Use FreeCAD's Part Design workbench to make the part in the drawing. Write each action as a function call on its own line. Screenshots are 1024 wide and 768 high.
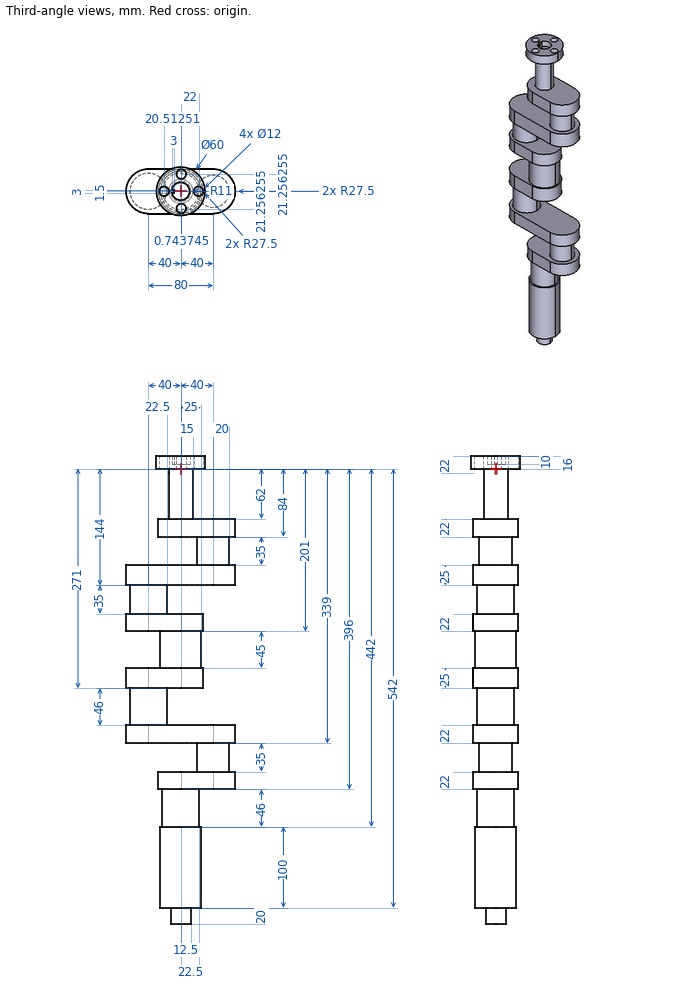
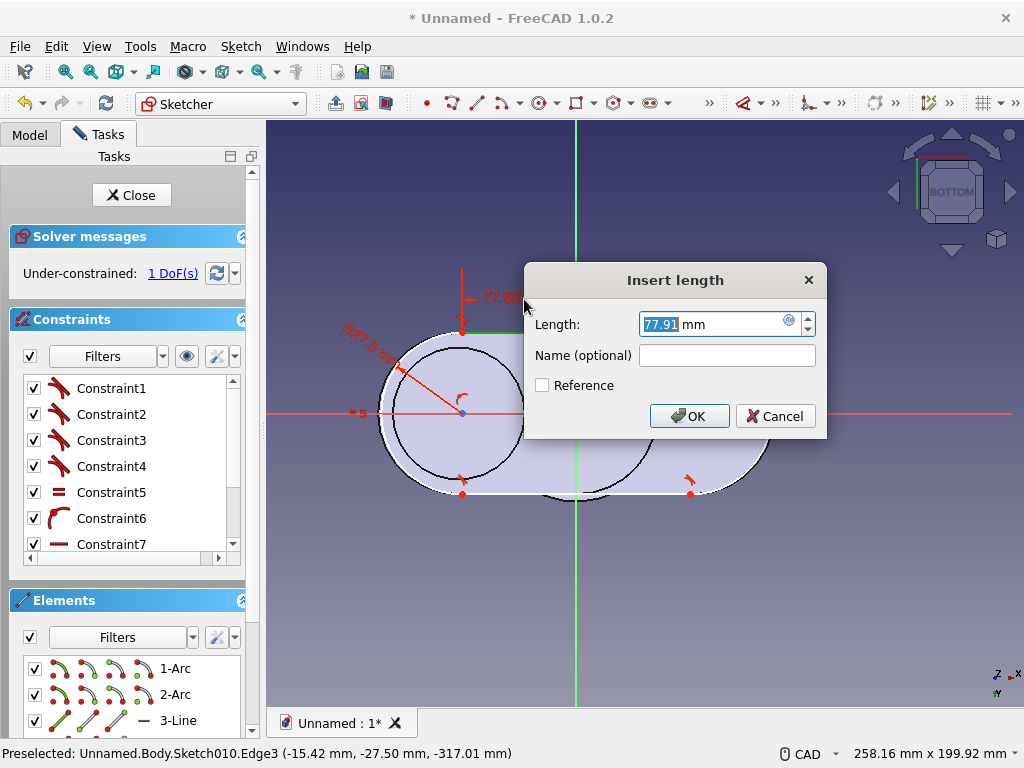
text(80)
key(Return)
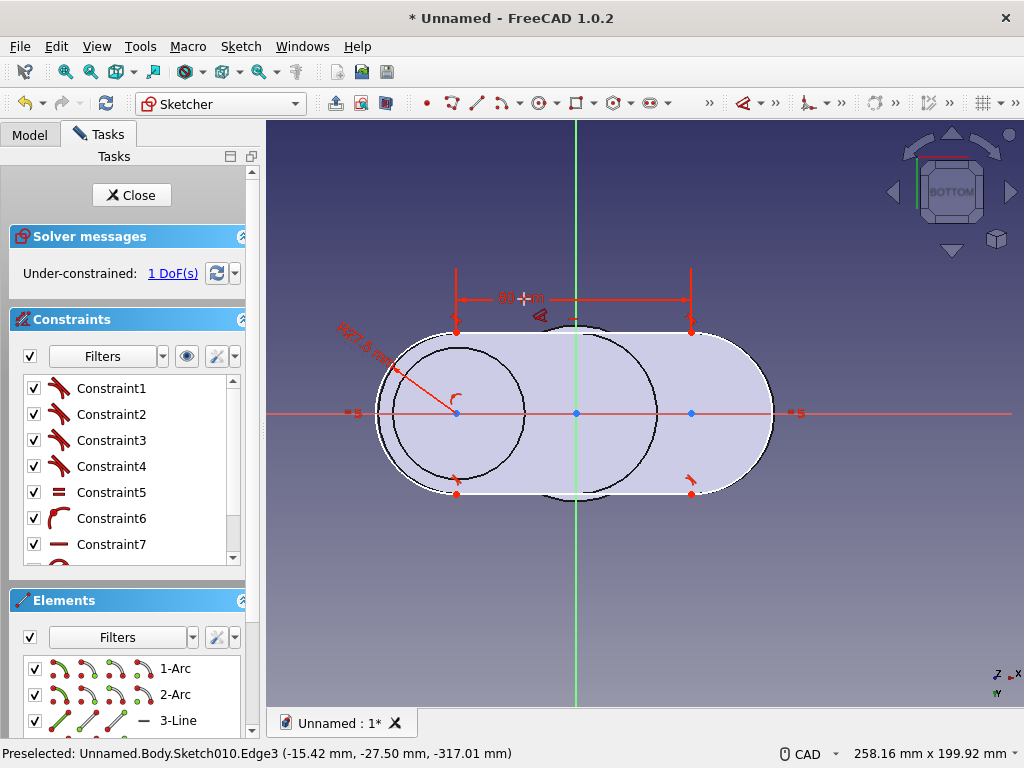
click(456, 333)
click(516, 447)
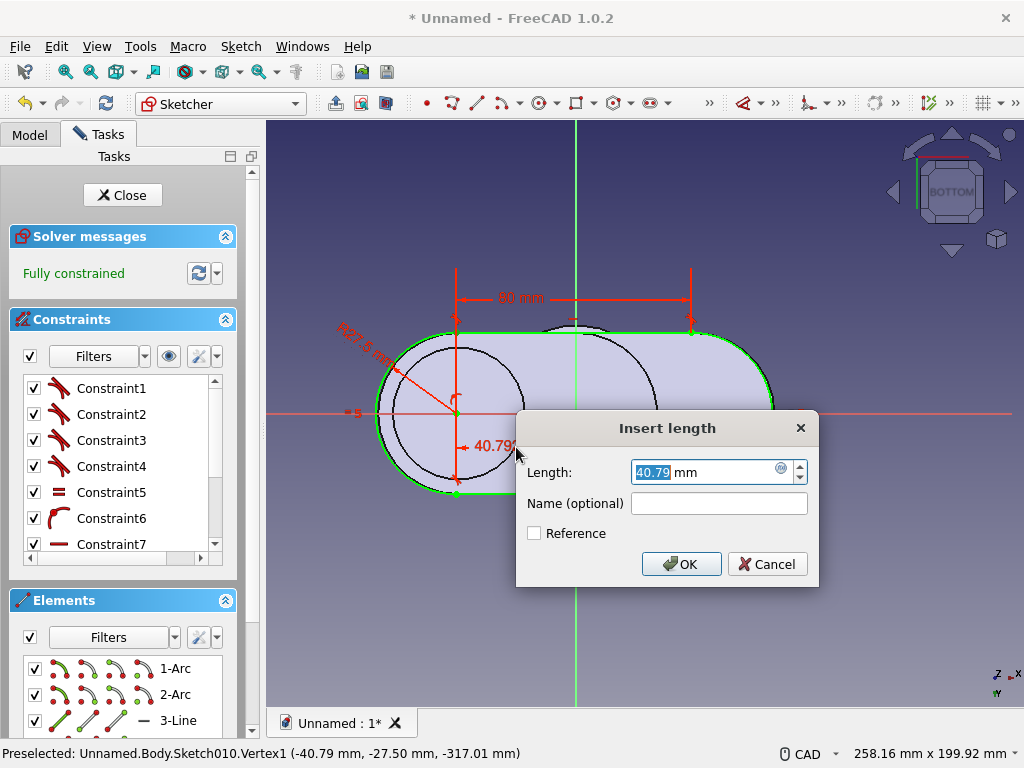
text(40)
key(Return)
key(Escape)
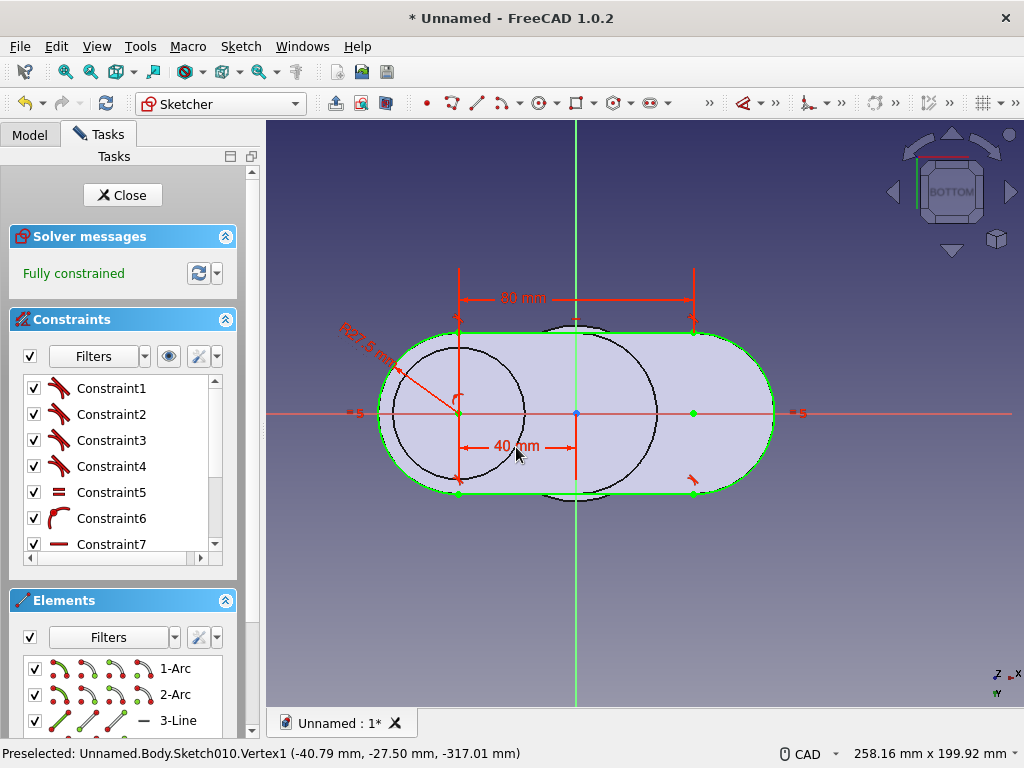
click(123, 195)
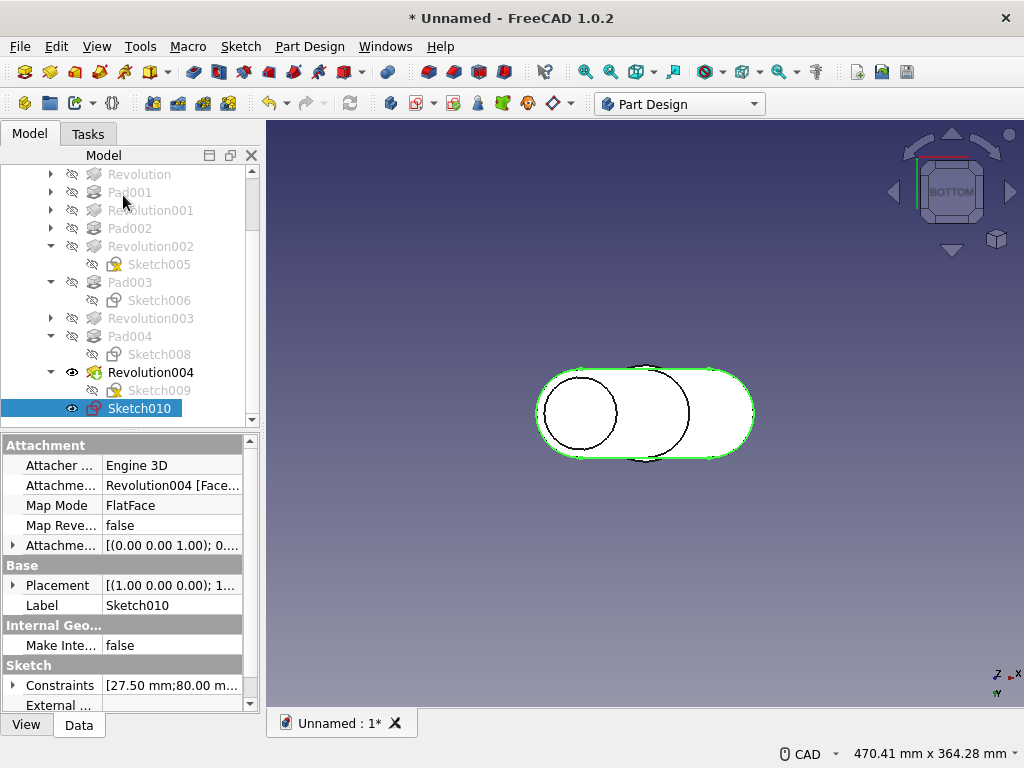
click(25, 72)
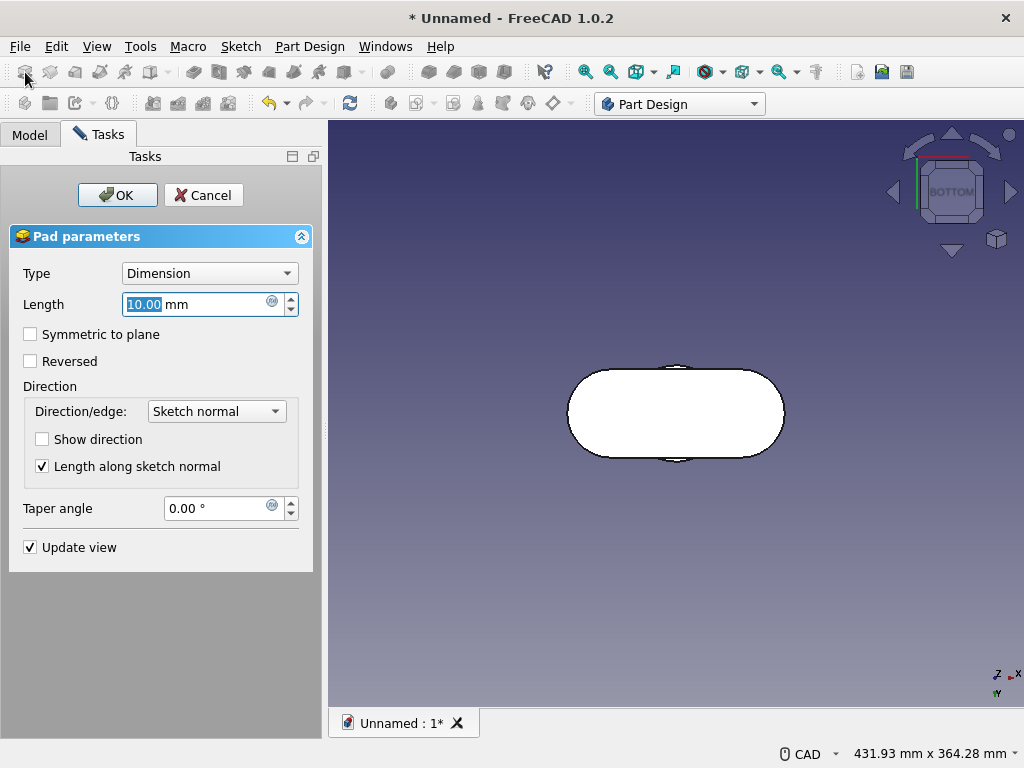
text(22)
key(Tab)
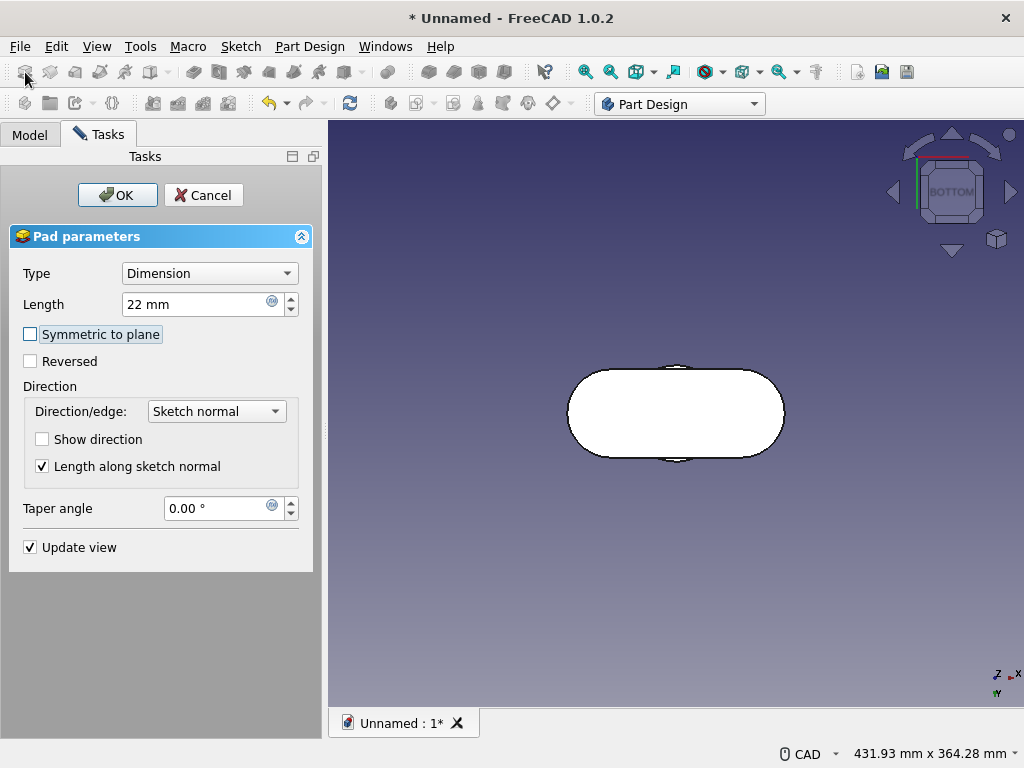
click(118, 195)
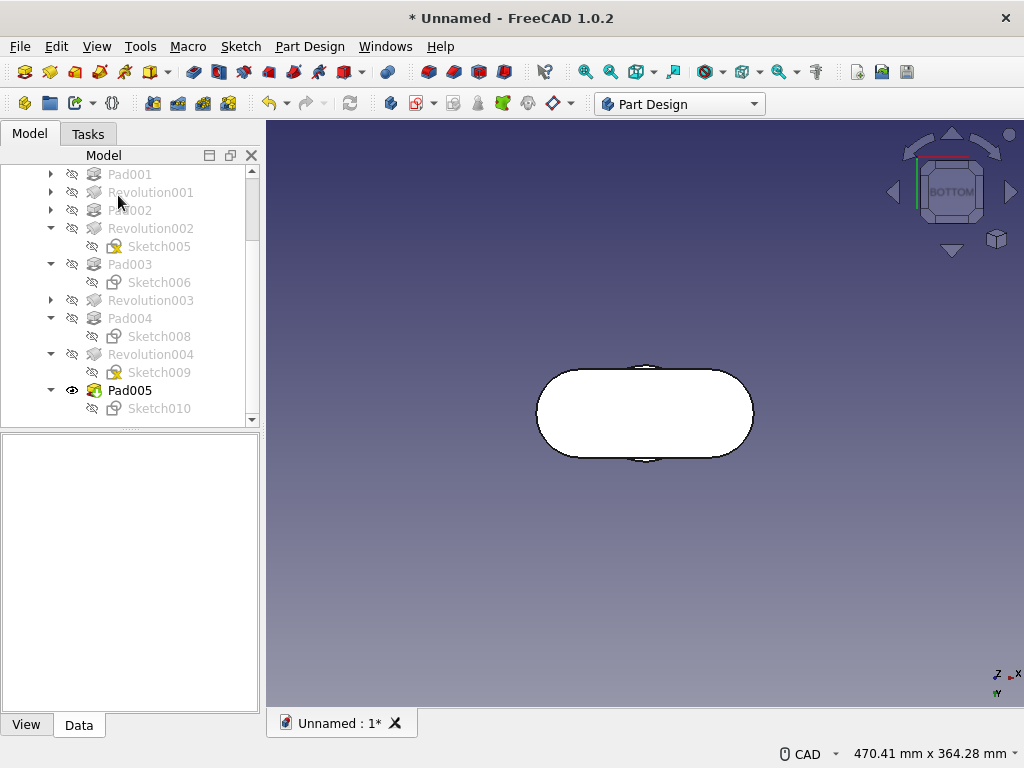
key(v)
key(f)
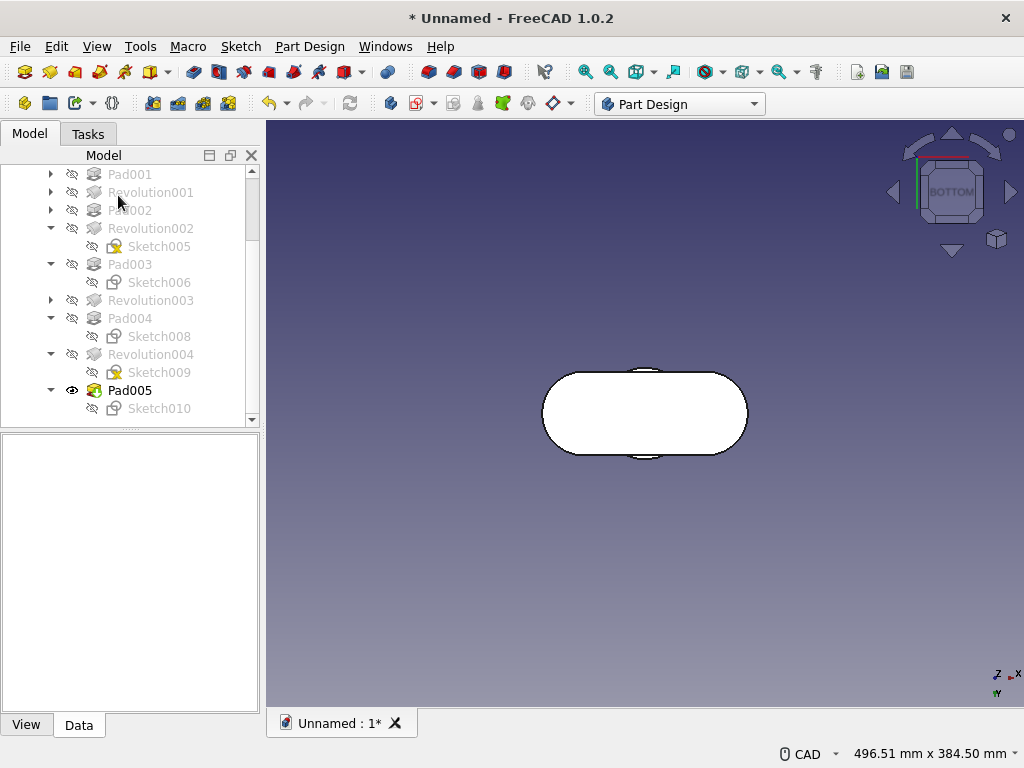
click(416, 104)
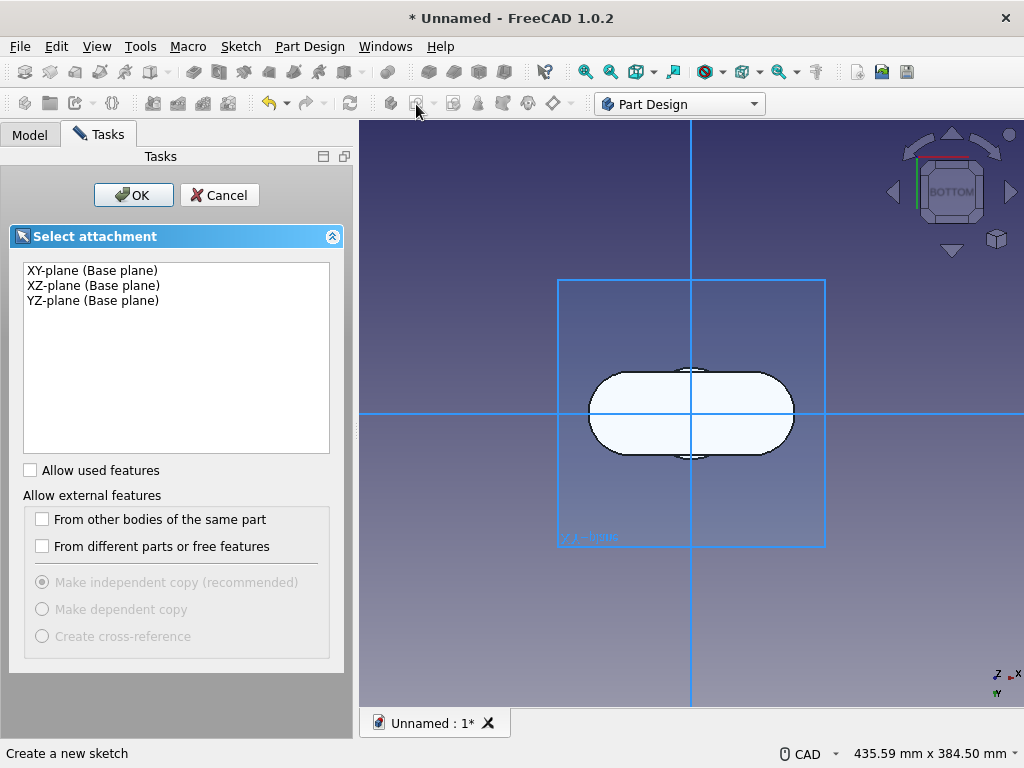
click(84, 286)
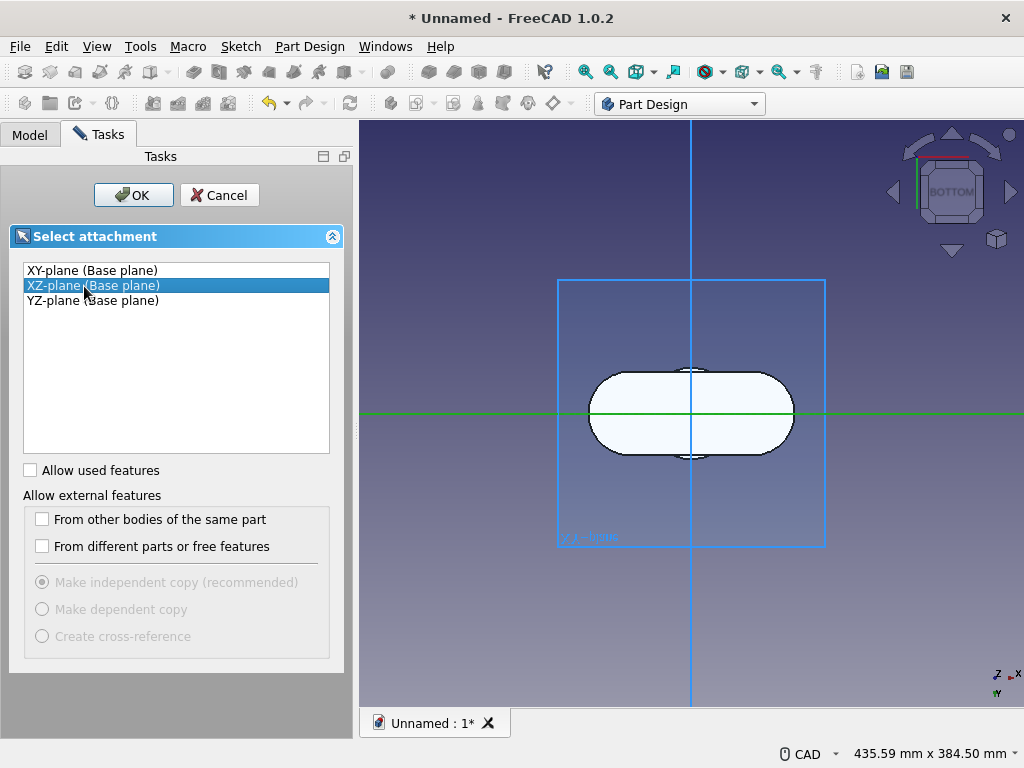
click(134, 195)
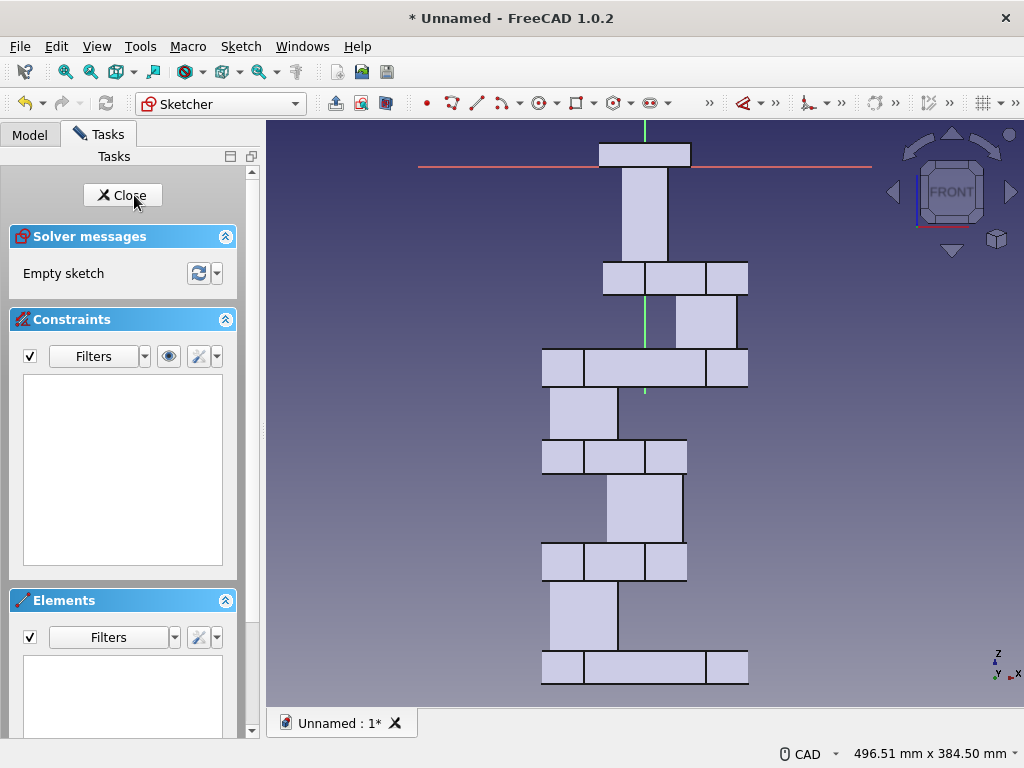
click(386, 104)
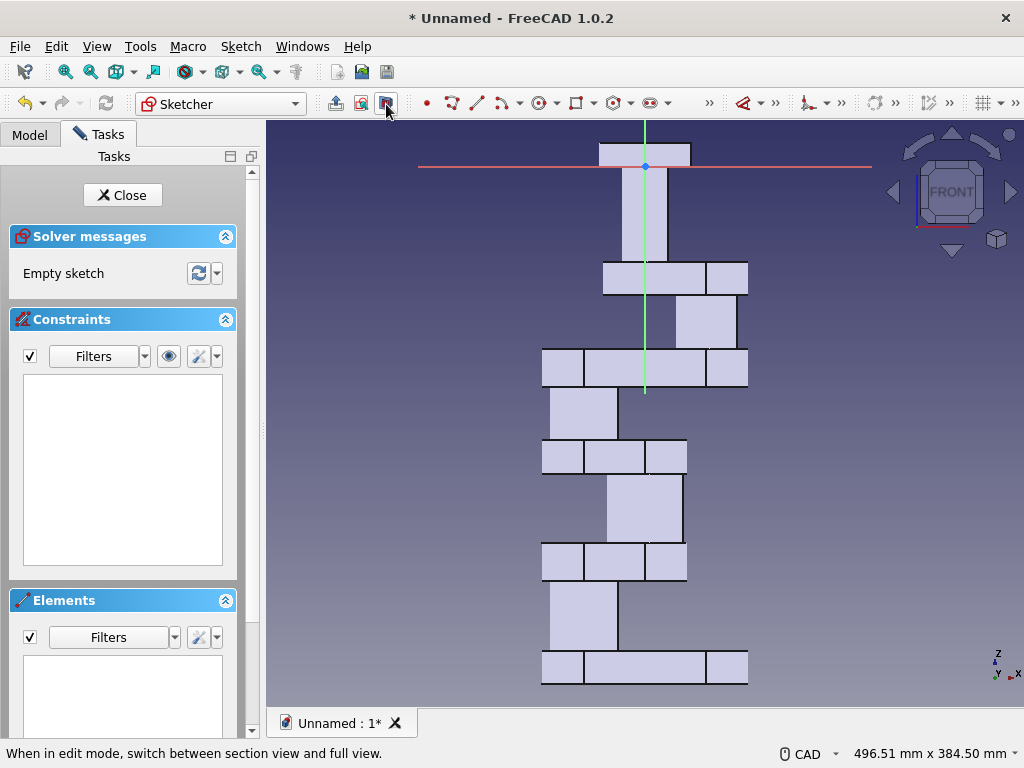
scroll(576, 414, down, 5)